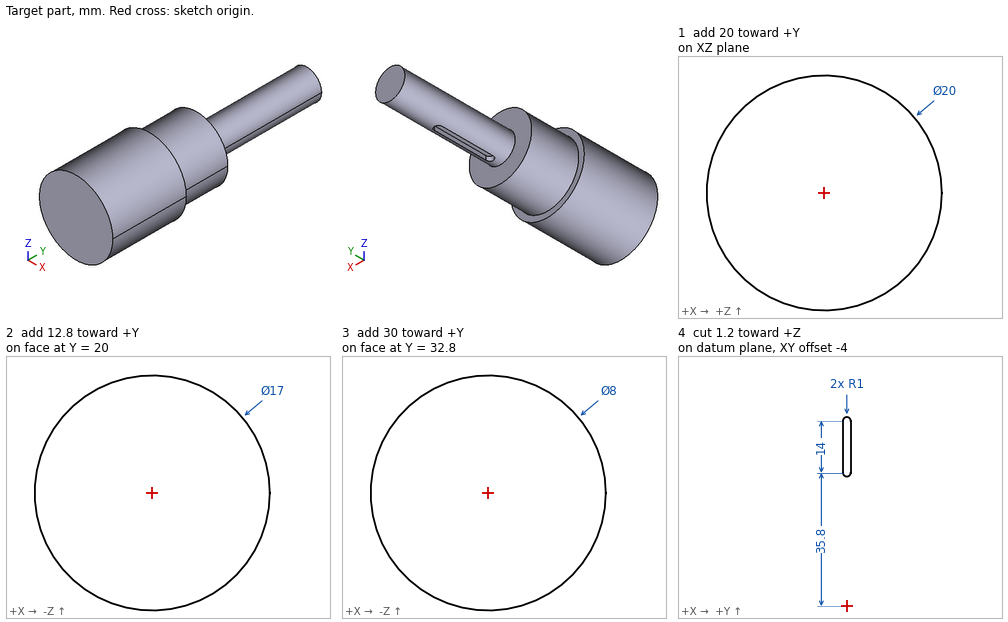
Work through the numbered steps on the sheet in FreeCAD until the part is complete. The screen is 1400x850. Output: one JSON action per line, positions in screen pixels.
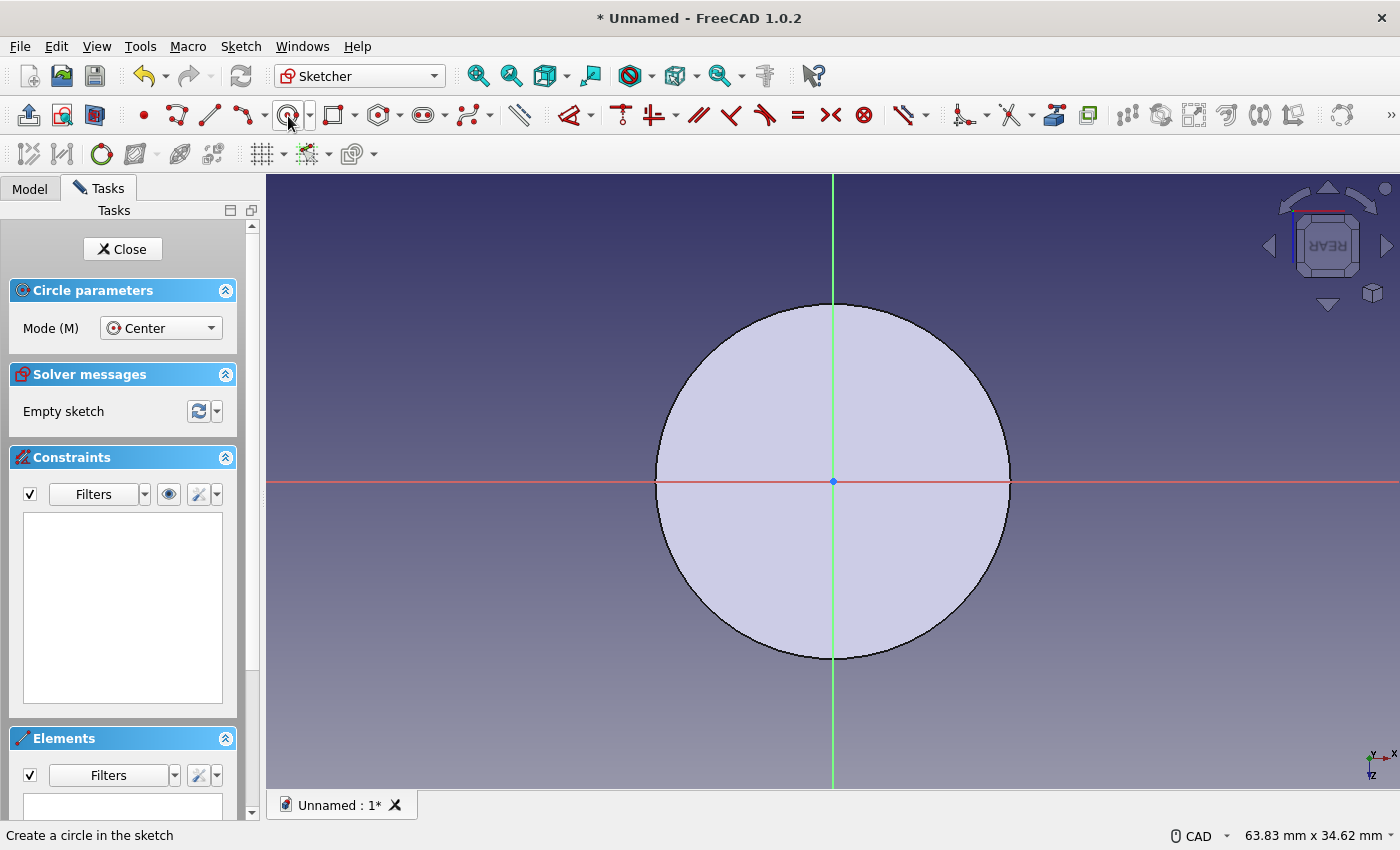
{"action": "left_click", "coordinate": [833, 482]}
{"action": "mouse_move", "coordinate": [940, 375]}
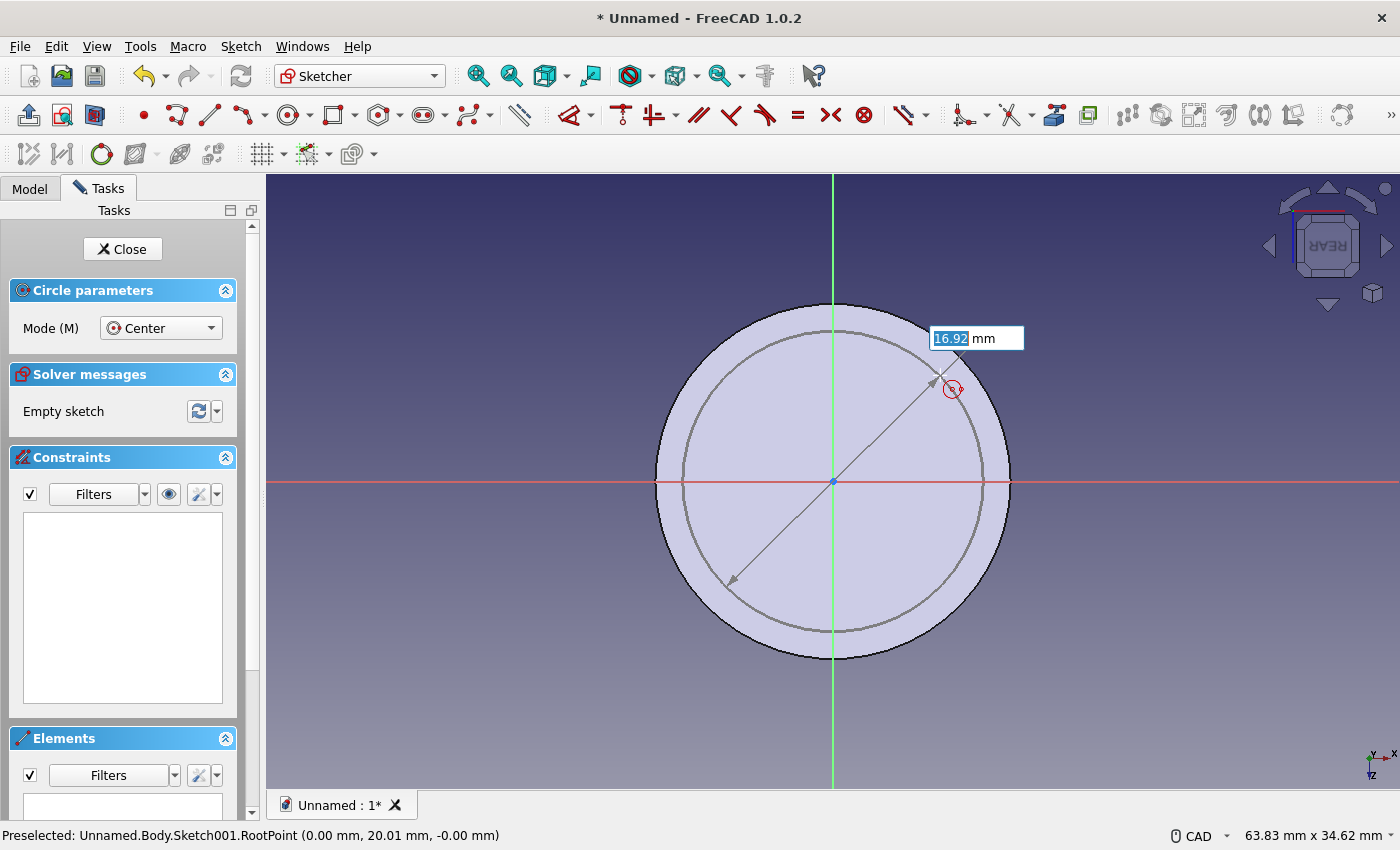
{"action": "type", "text": "17"}
{"action": "key", "text": "Return"}
{"action": "key", "text": "Escape"}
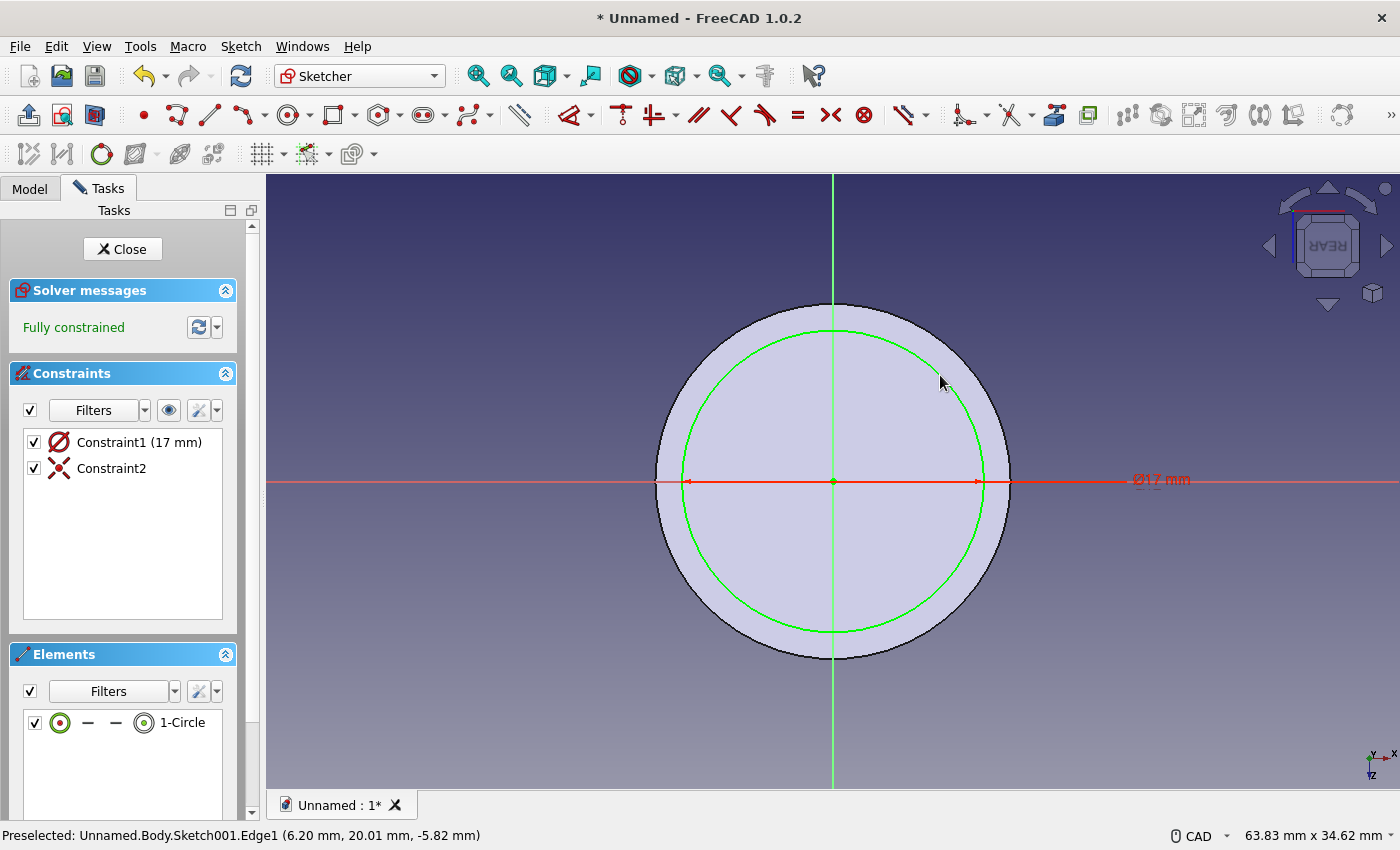
{"action": "left_click", "coordinate": [123, 249]}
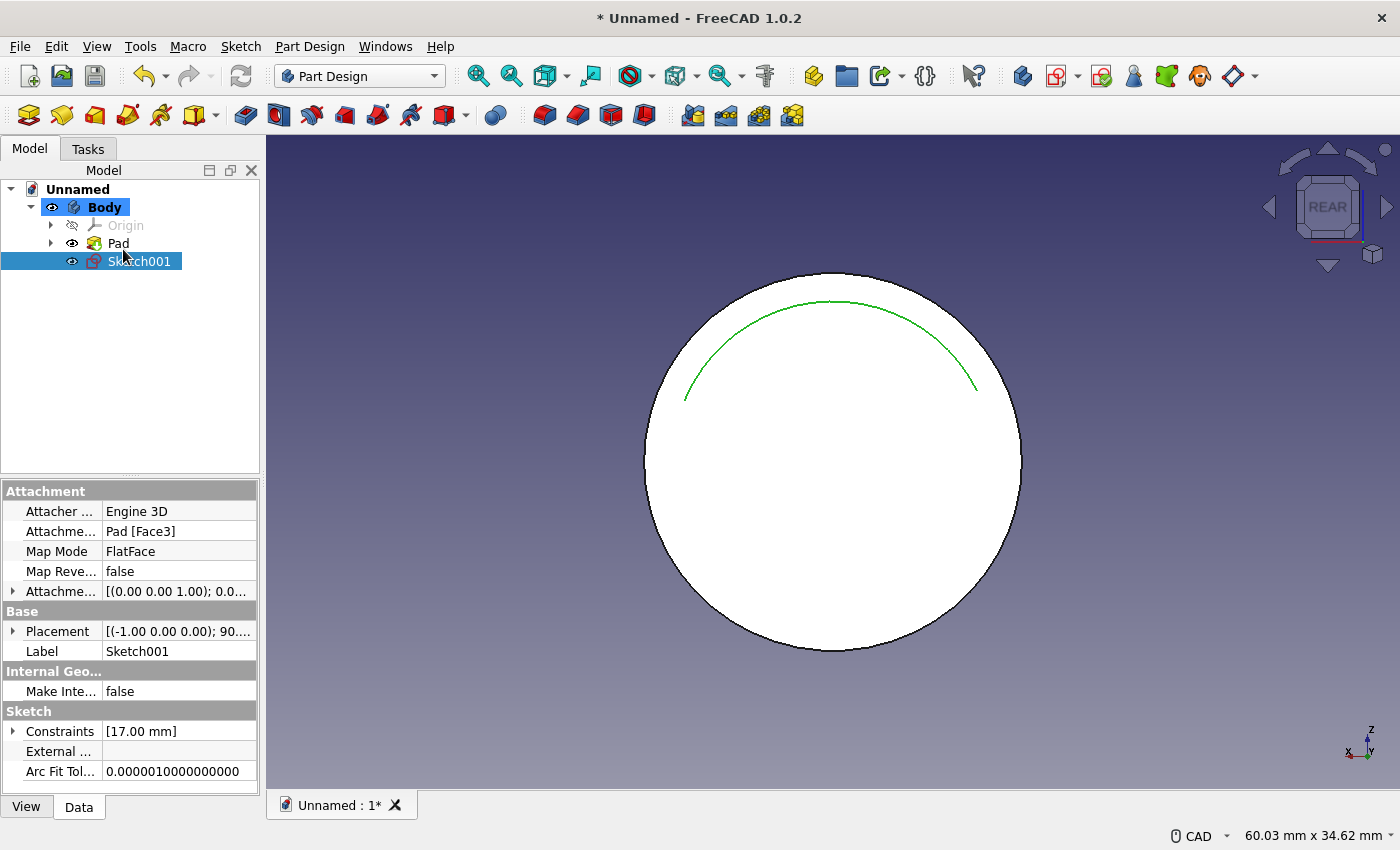
{"action": "left_click", "coordinate": [29, 116]}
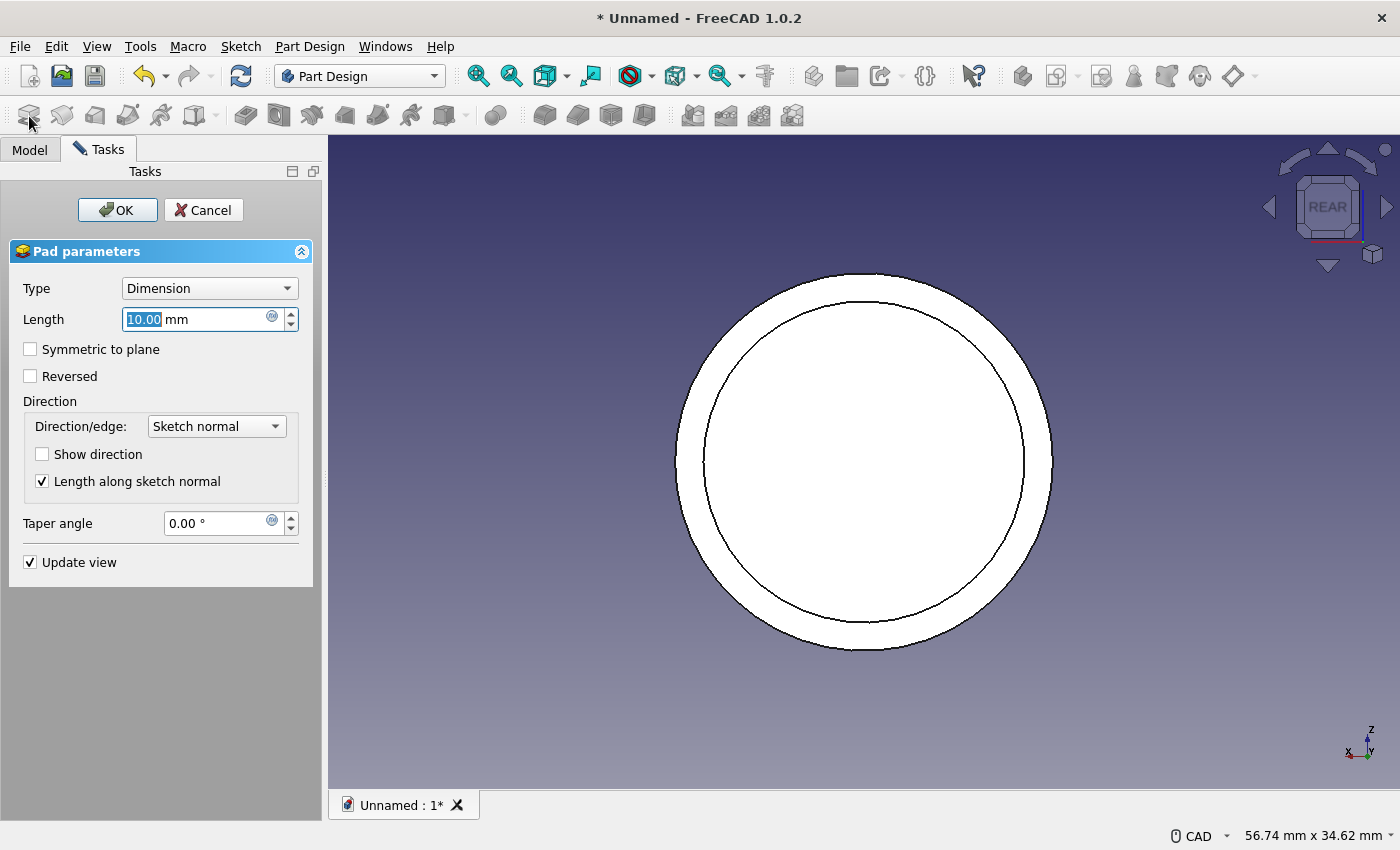
{"action": "type", "text": "12.8"}
{"action": "key", "text": "Tab"}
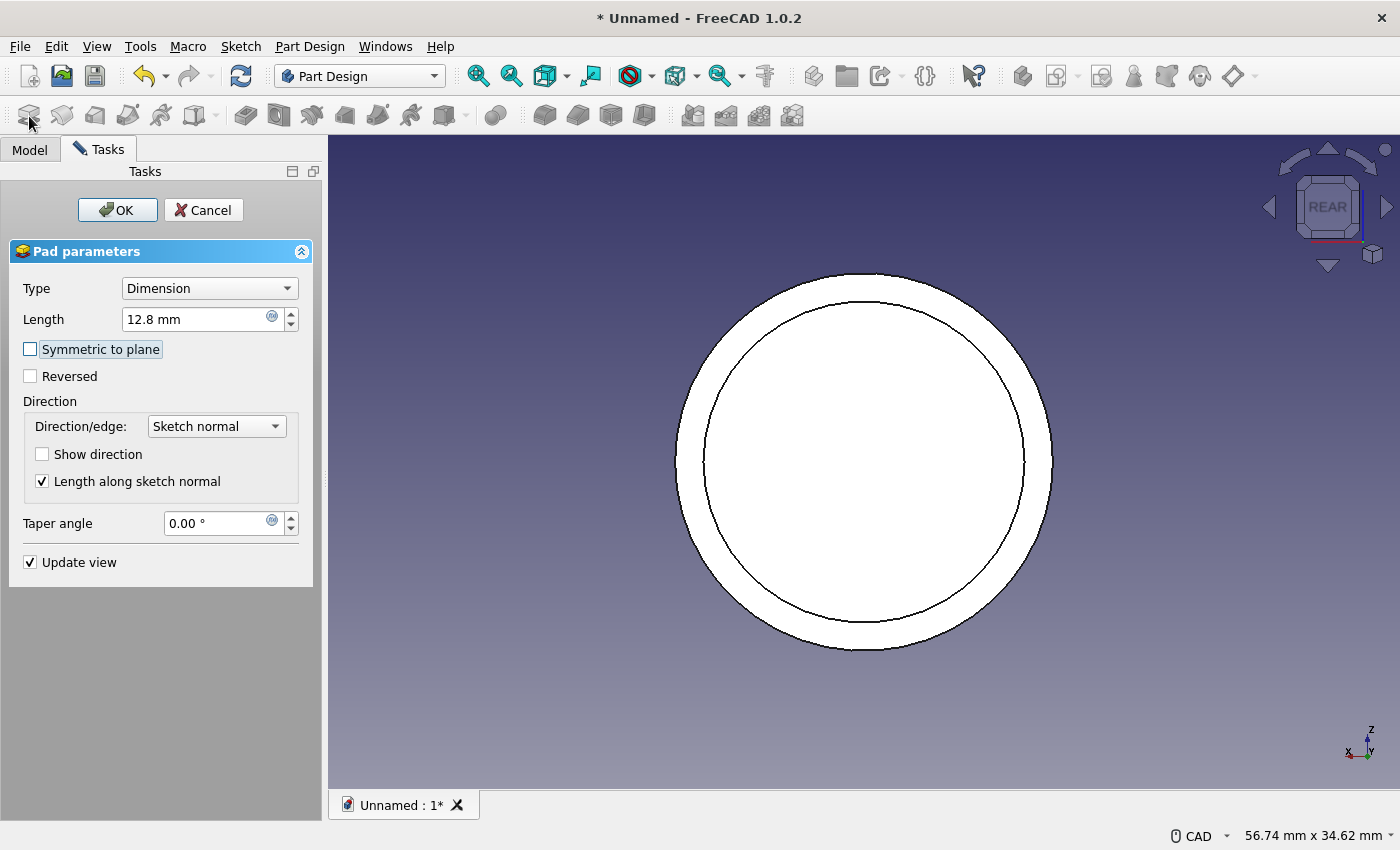
{"action": "left_click", "coordinate": [118, 210]}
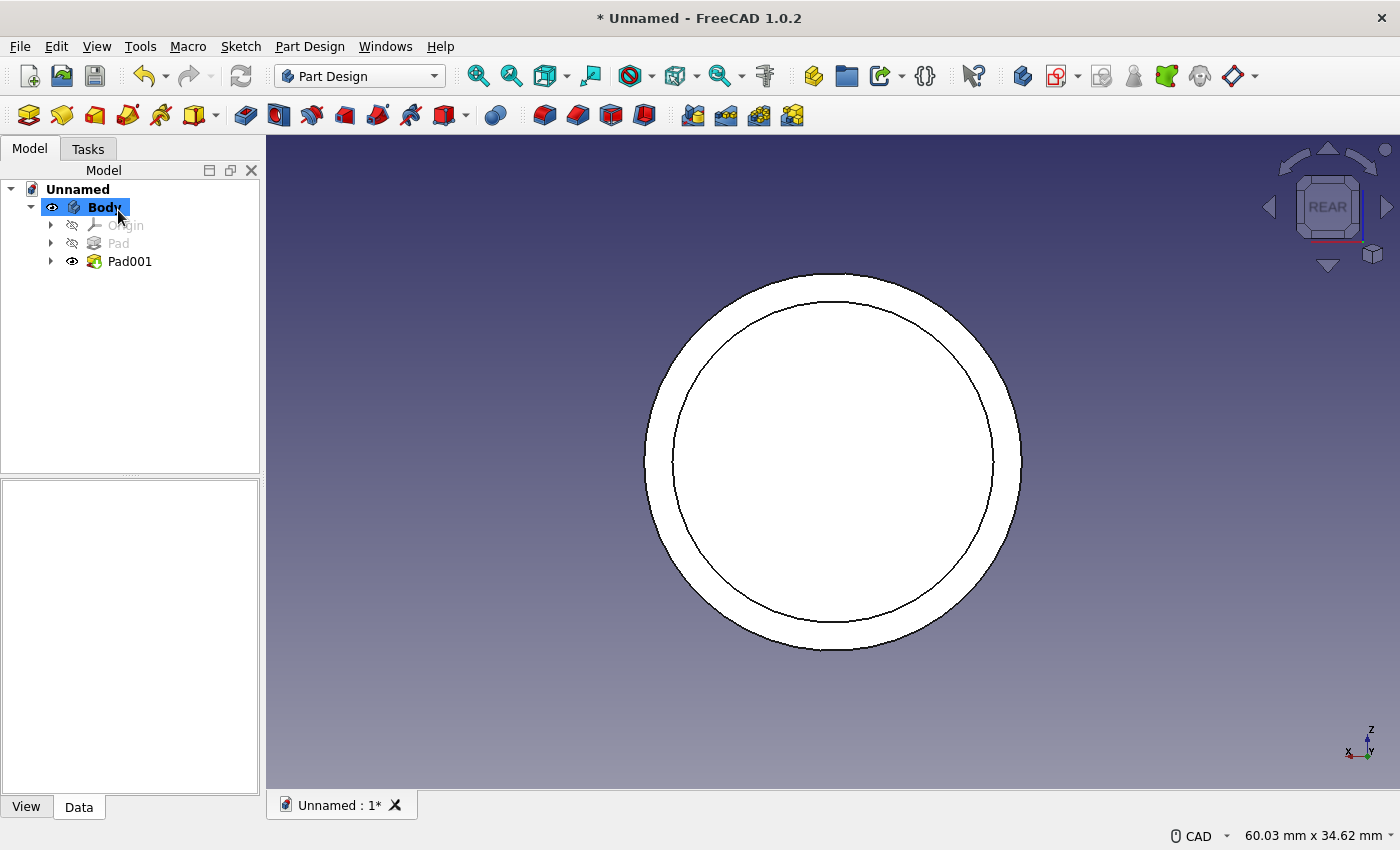
{"action": "left_click", "coordinate": [833, 461]}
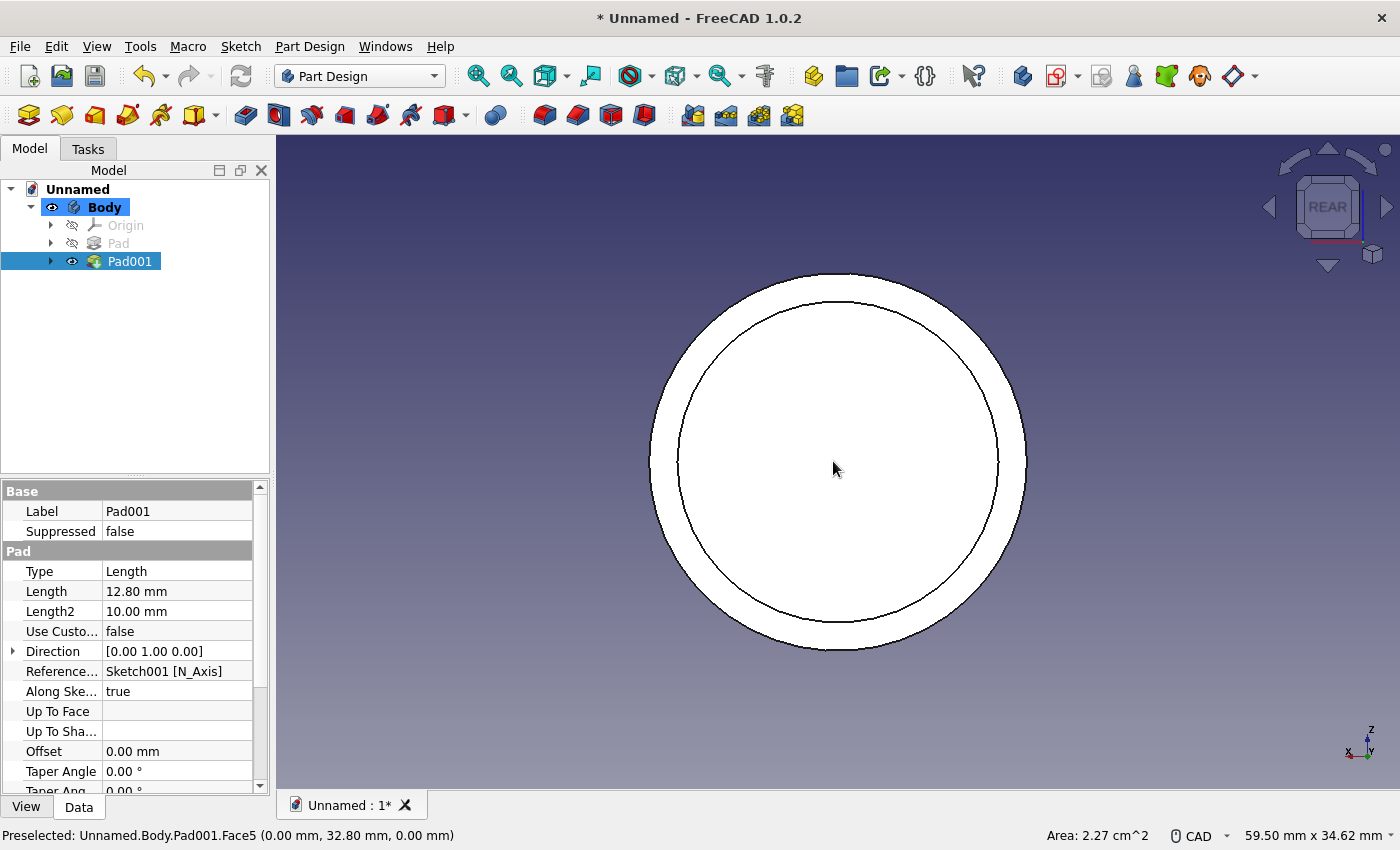
{"action": "left_click", "coordinate": [1056, 76]}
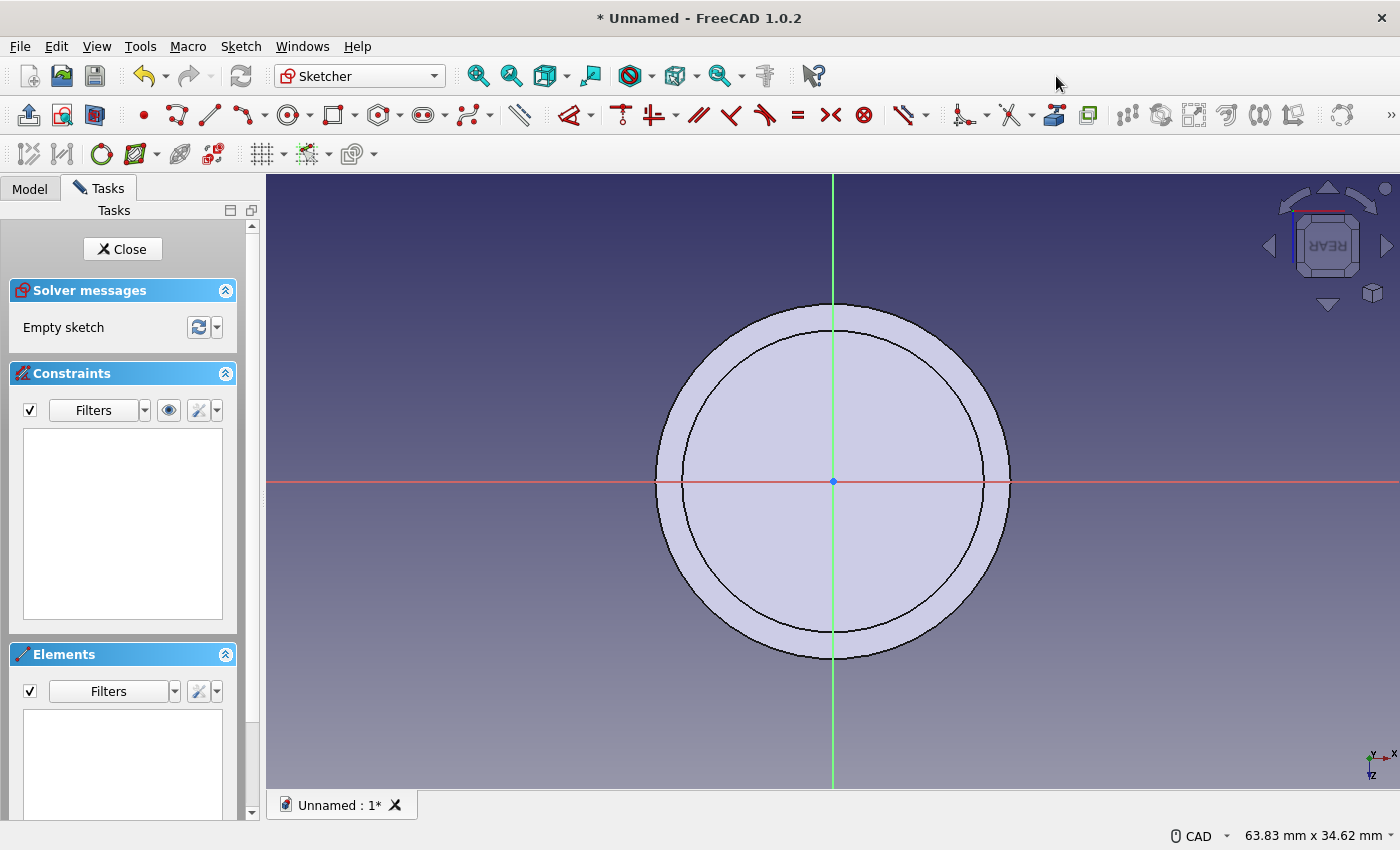
{"action": "scroll", "coordinate": [873, 481], "scroll_direction": "up", "scroll_amount": 5}